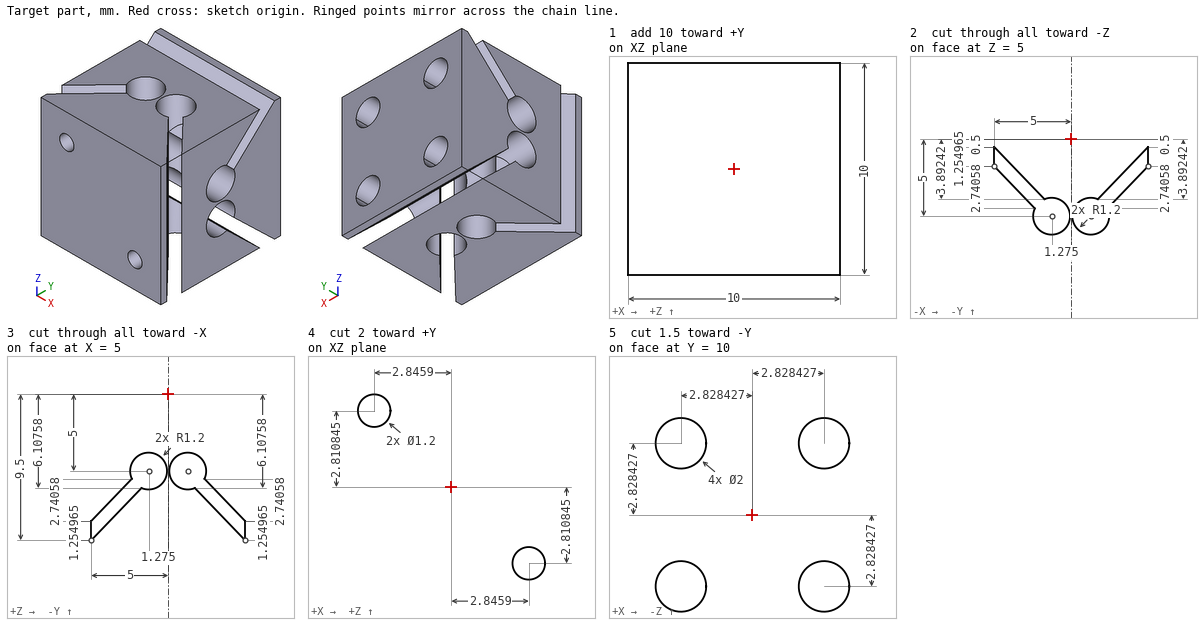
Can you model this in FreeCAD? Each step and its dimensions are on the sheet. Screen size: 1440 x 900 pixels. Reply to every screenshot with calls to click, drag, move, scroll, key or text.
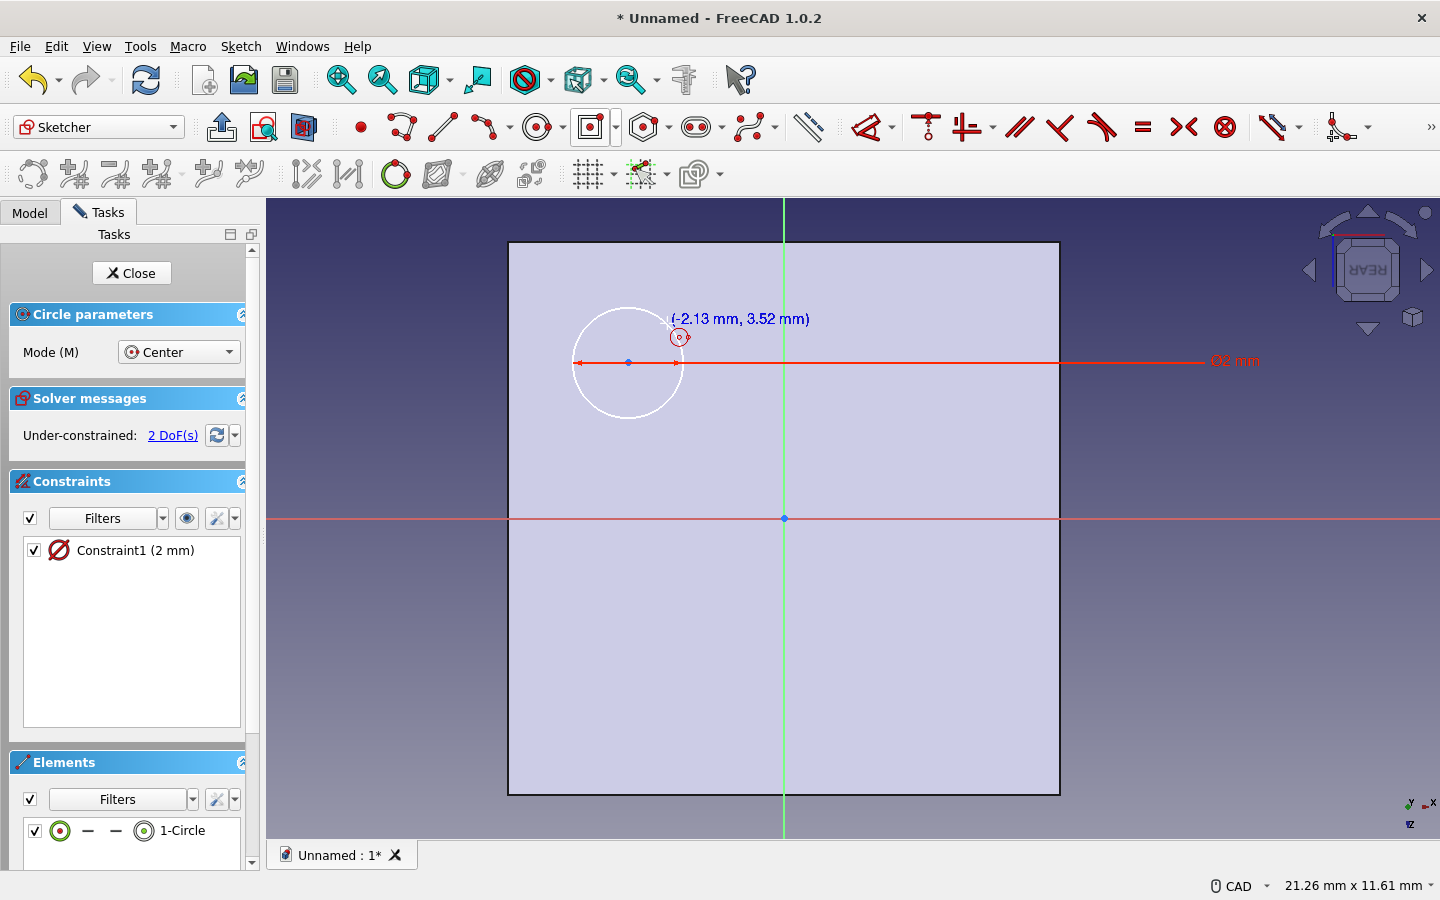
click(940, 362)
move(980, 323)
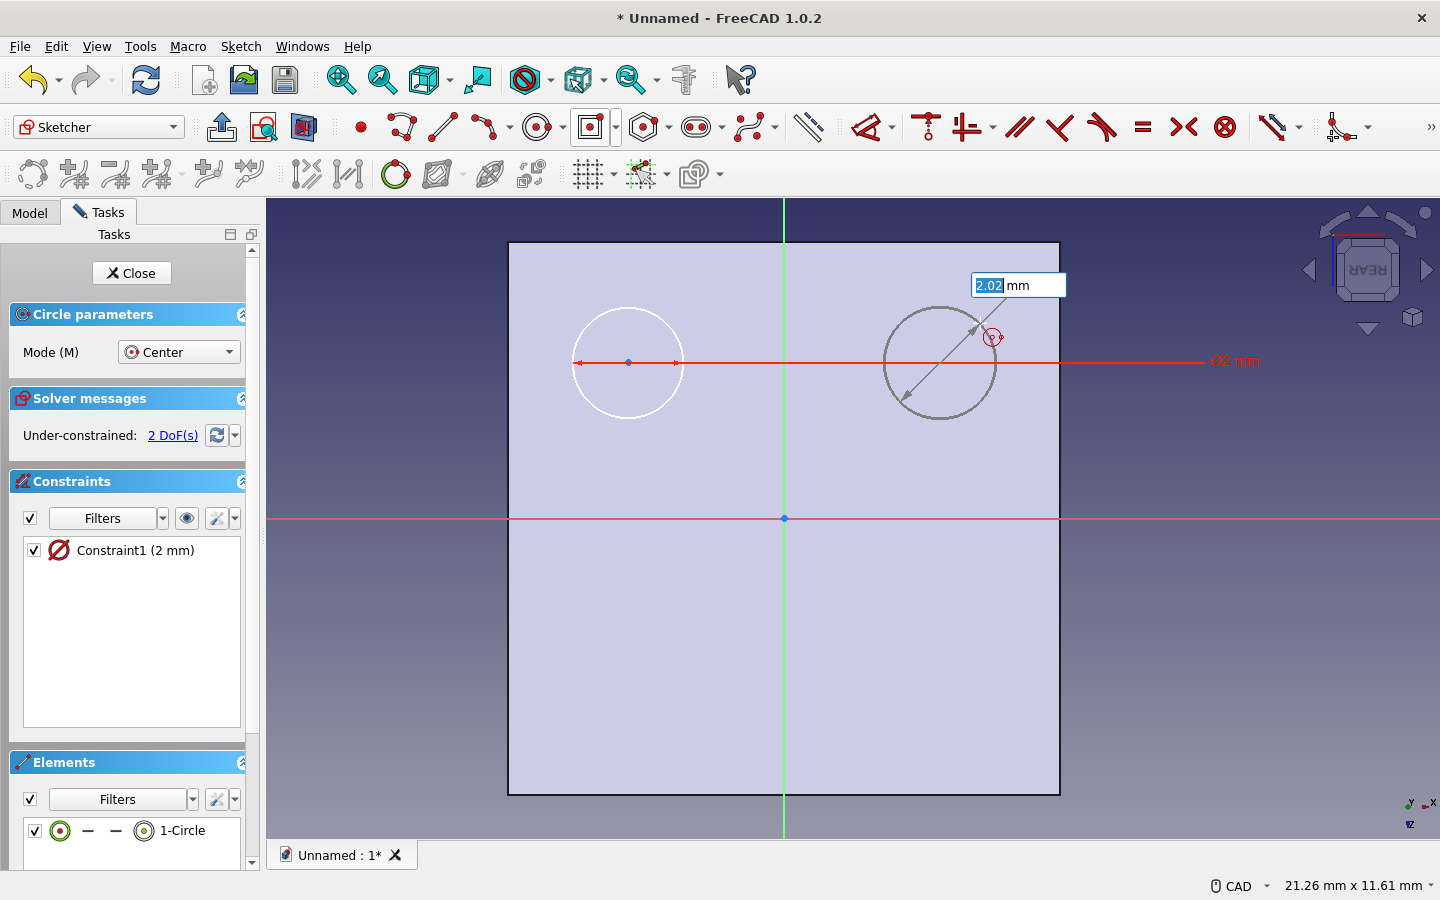
text(2)
key(Return)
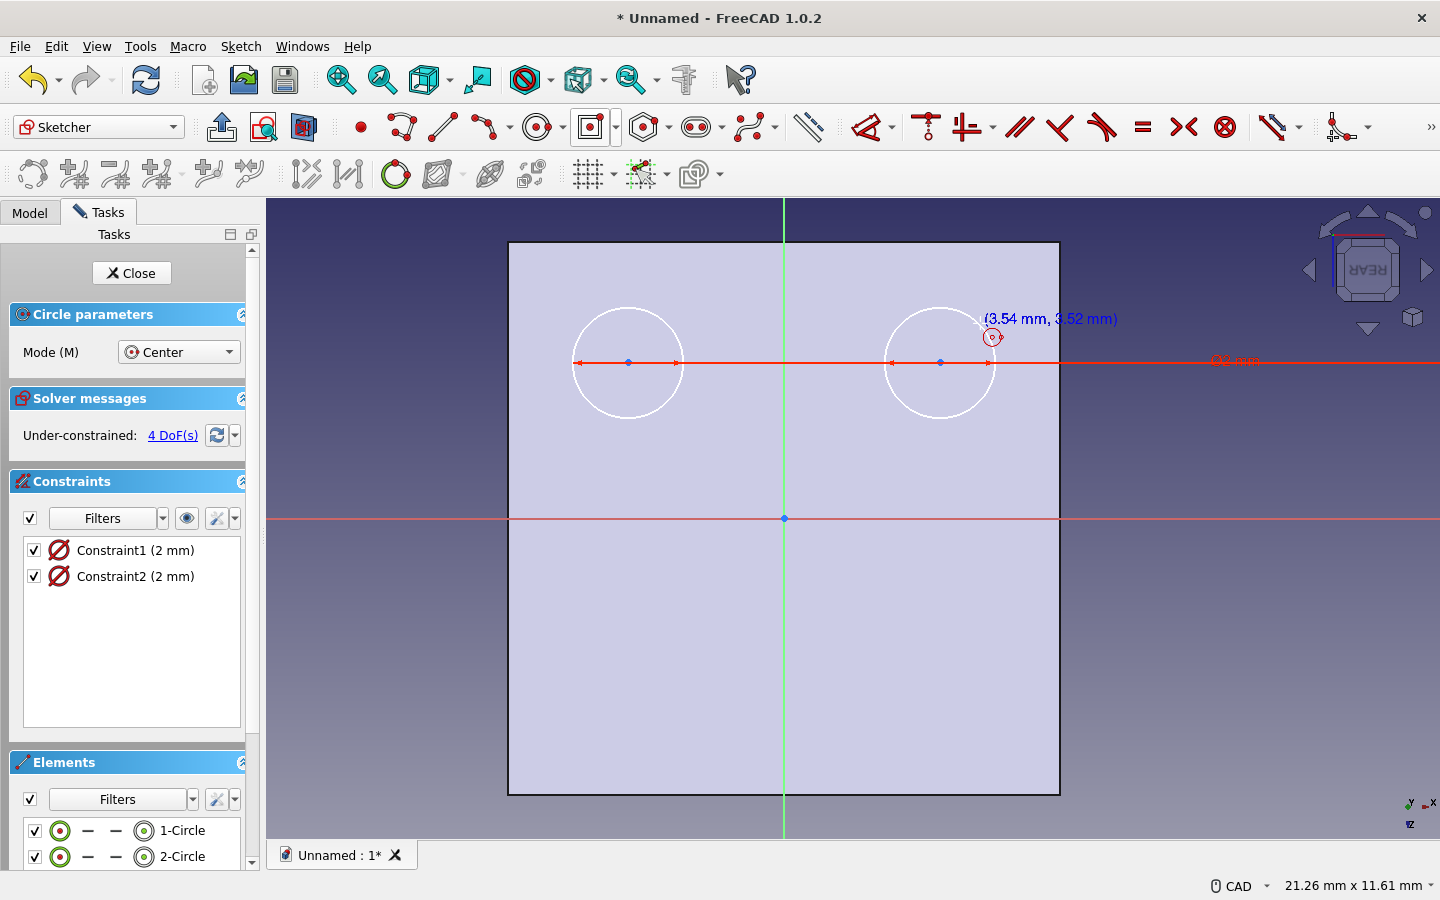
click(940, 675)
move(980, 636)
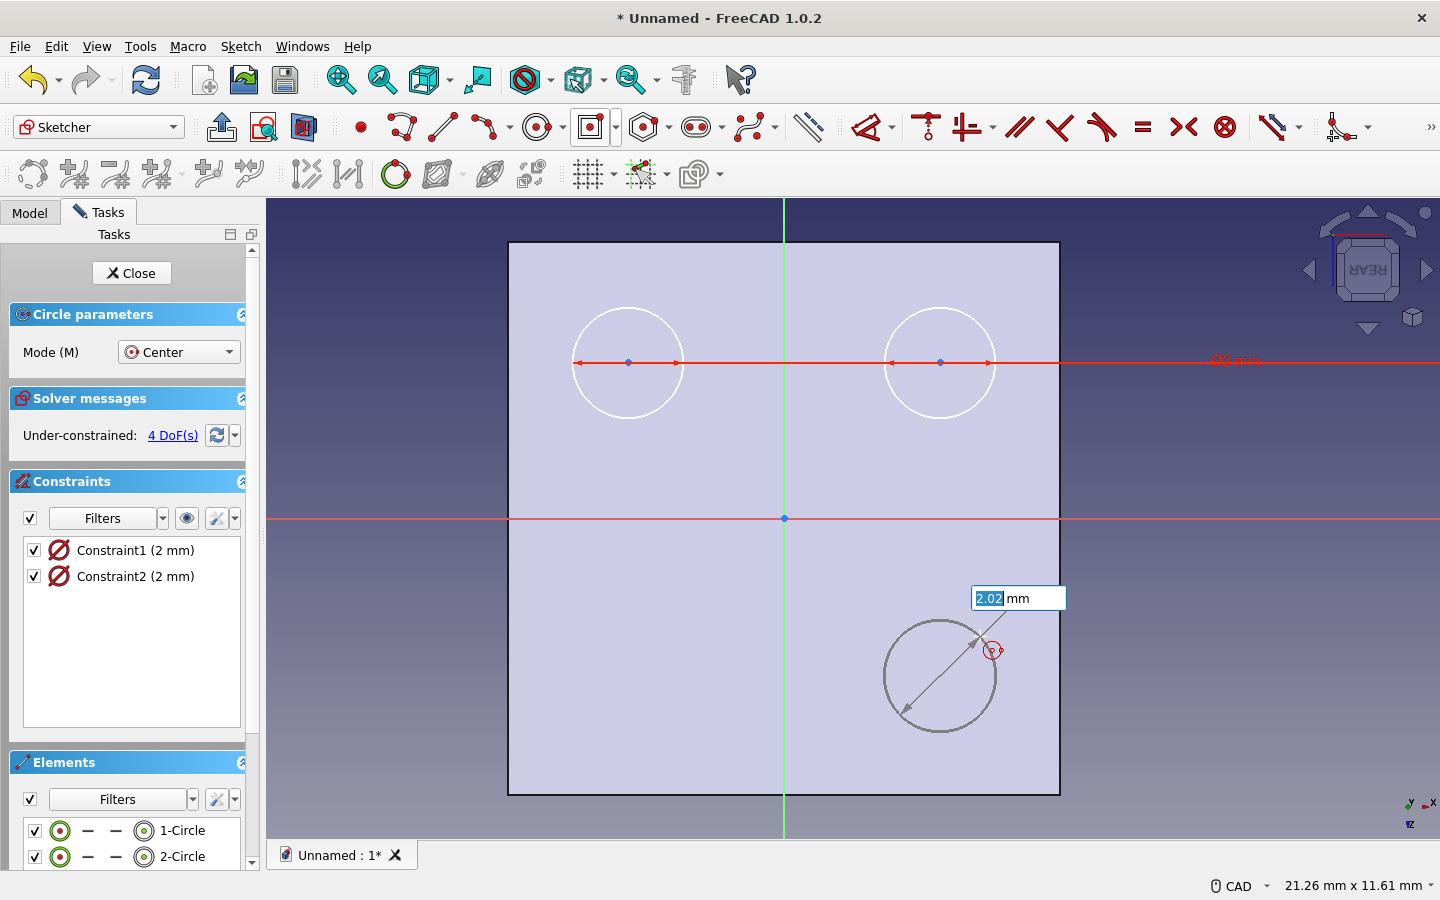
text(2)
key(Return)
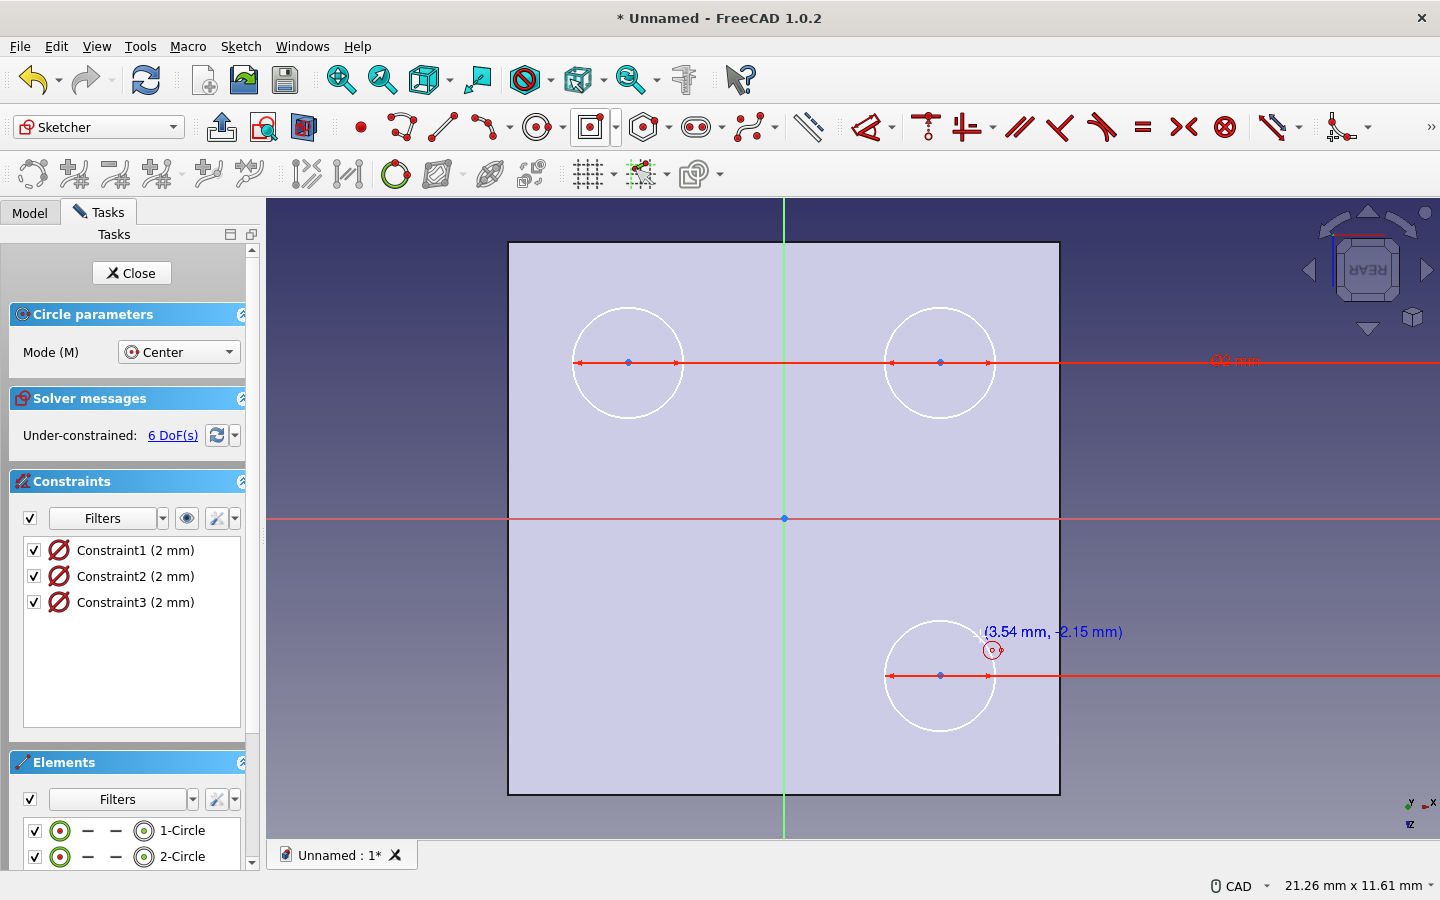
click(628, 675)
move(667, 636)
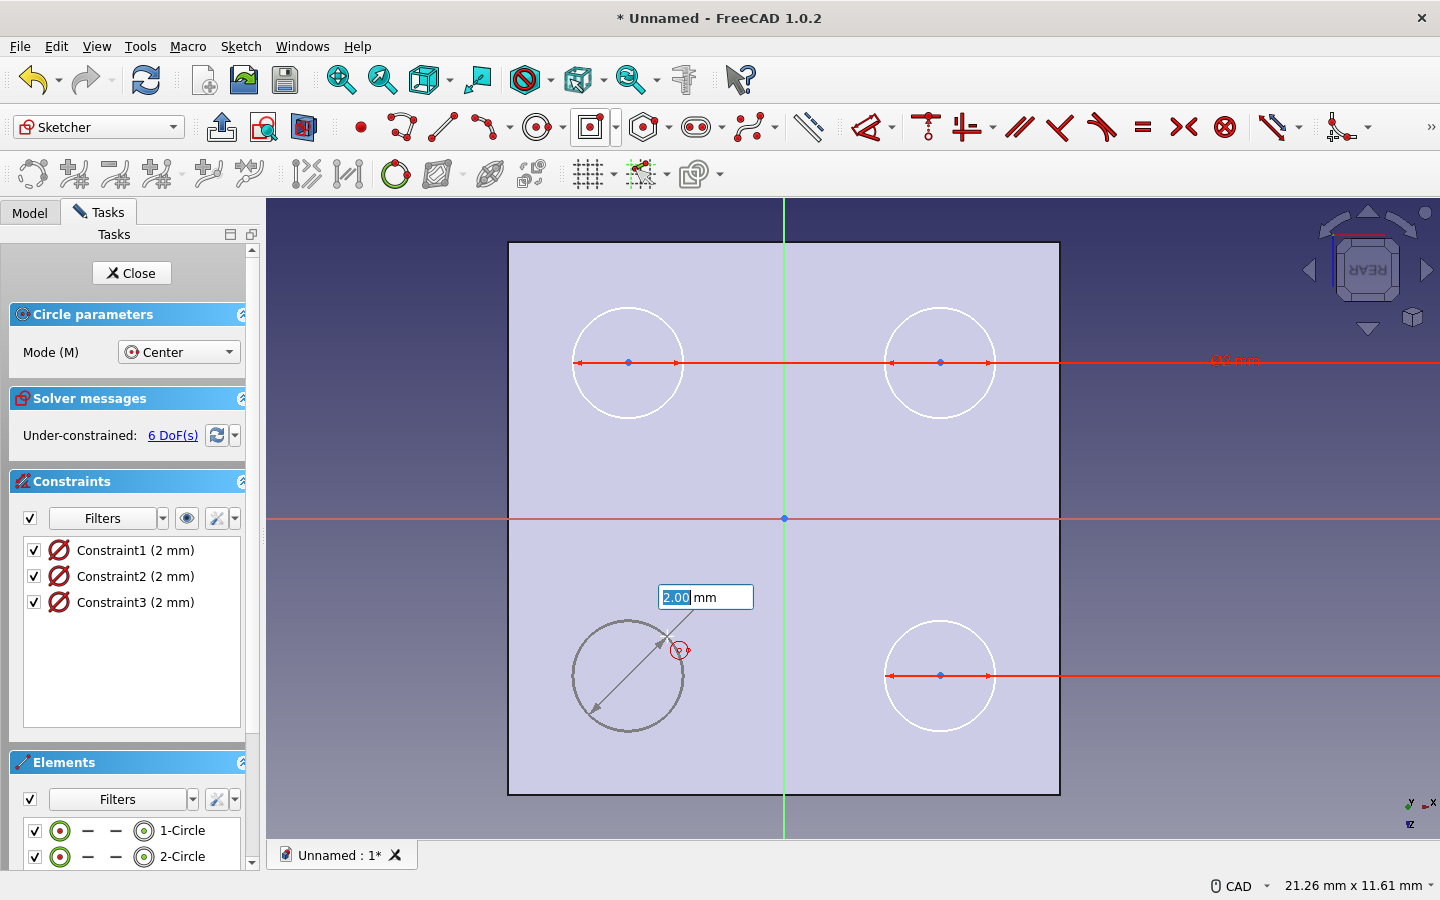
text(2)
key(Return)
key(Escape)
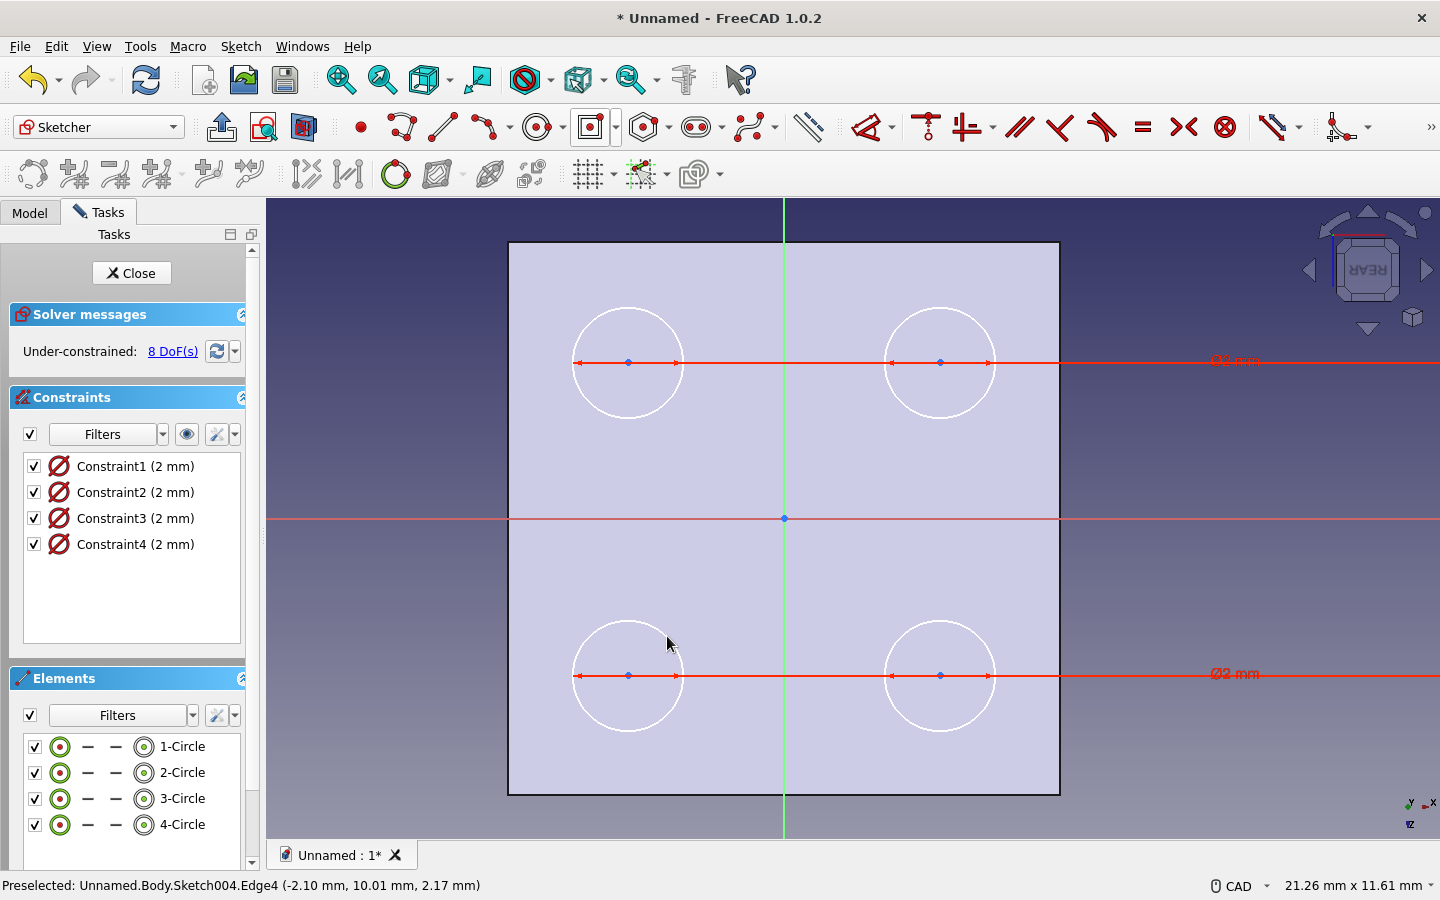
click(628, 363)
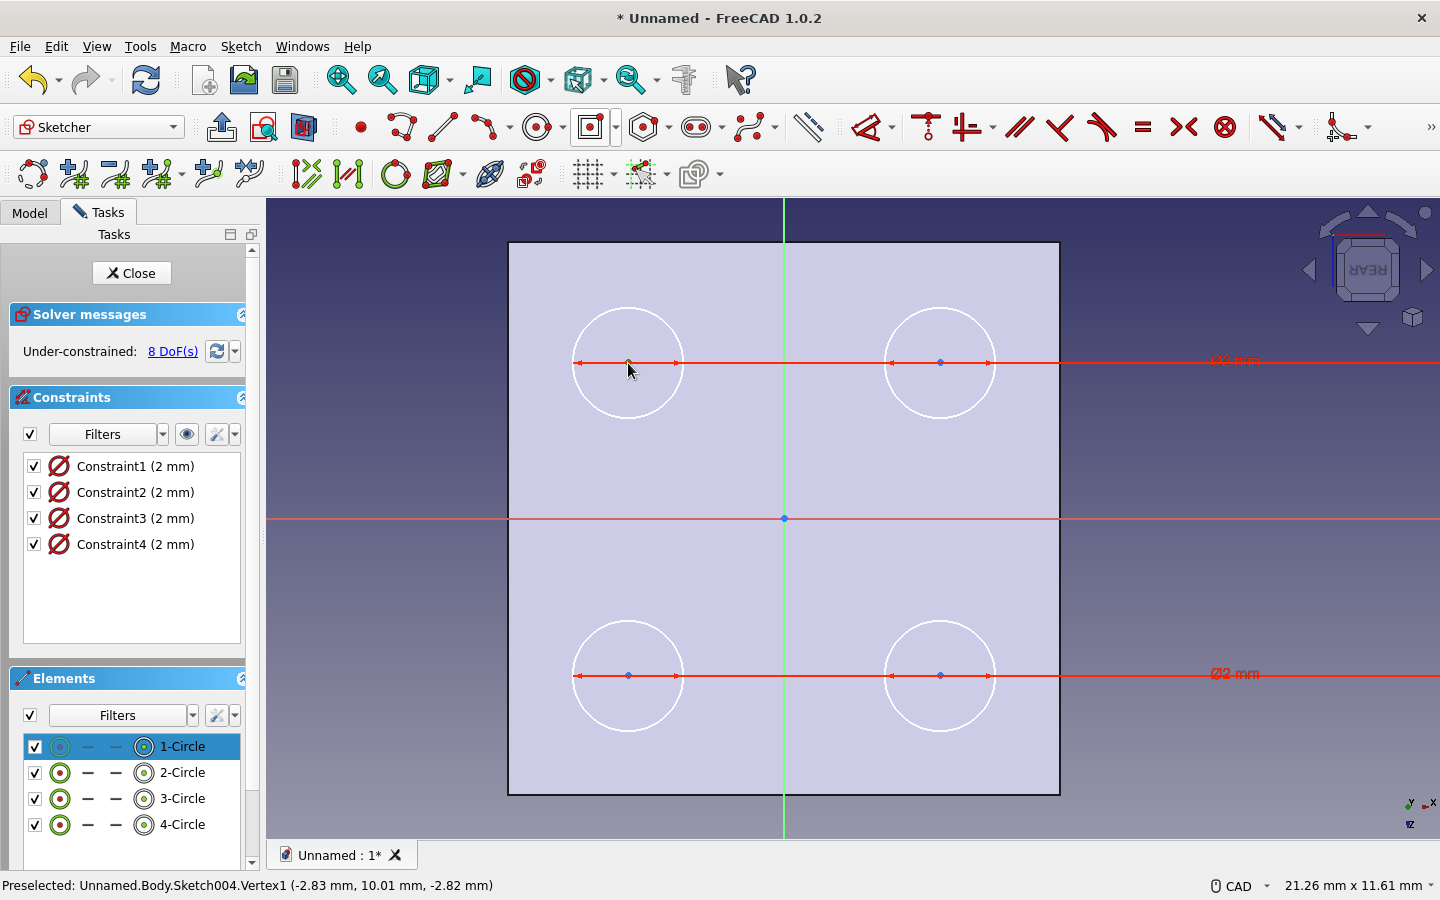
click(940, 363)